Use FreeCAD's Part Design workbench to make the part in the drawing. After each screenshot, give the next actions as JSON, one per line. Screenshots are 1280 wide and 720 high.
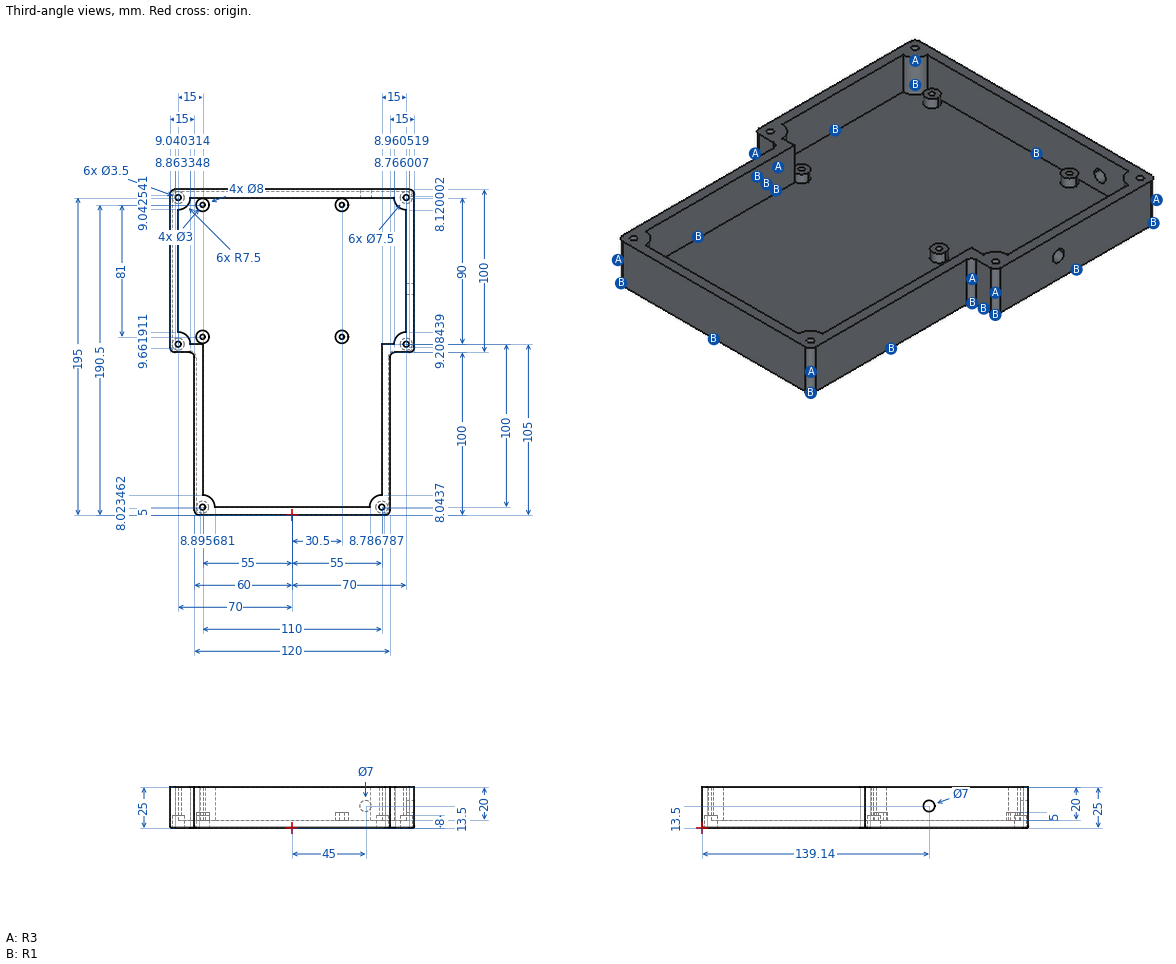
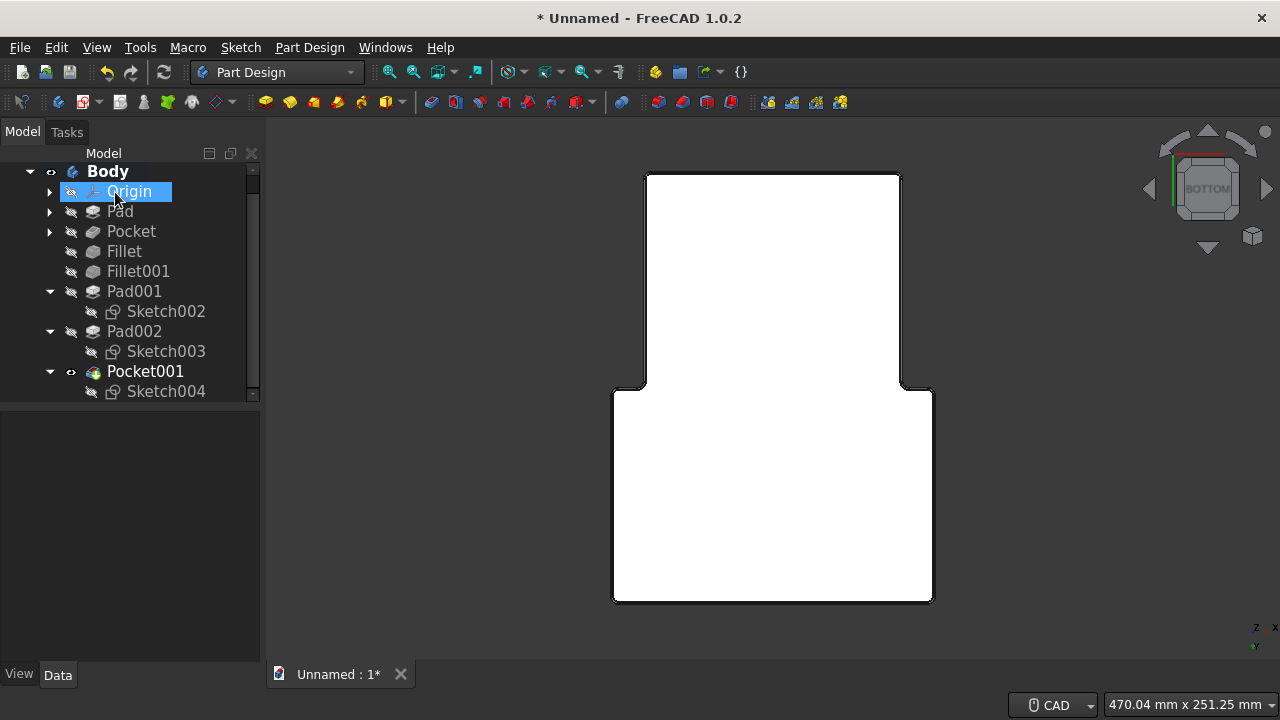
{"action": "left_click", "coordinate": [773, 448]}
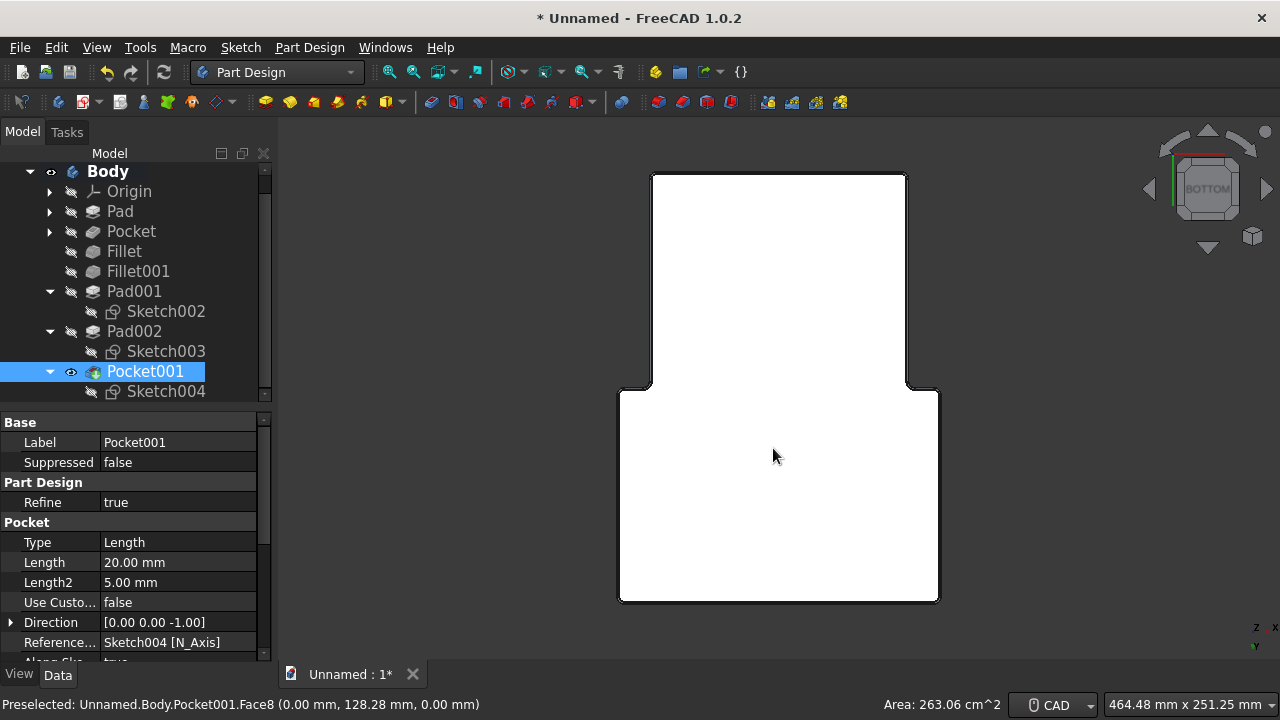
{"action": "left_click", "coordinate": [84, 102]}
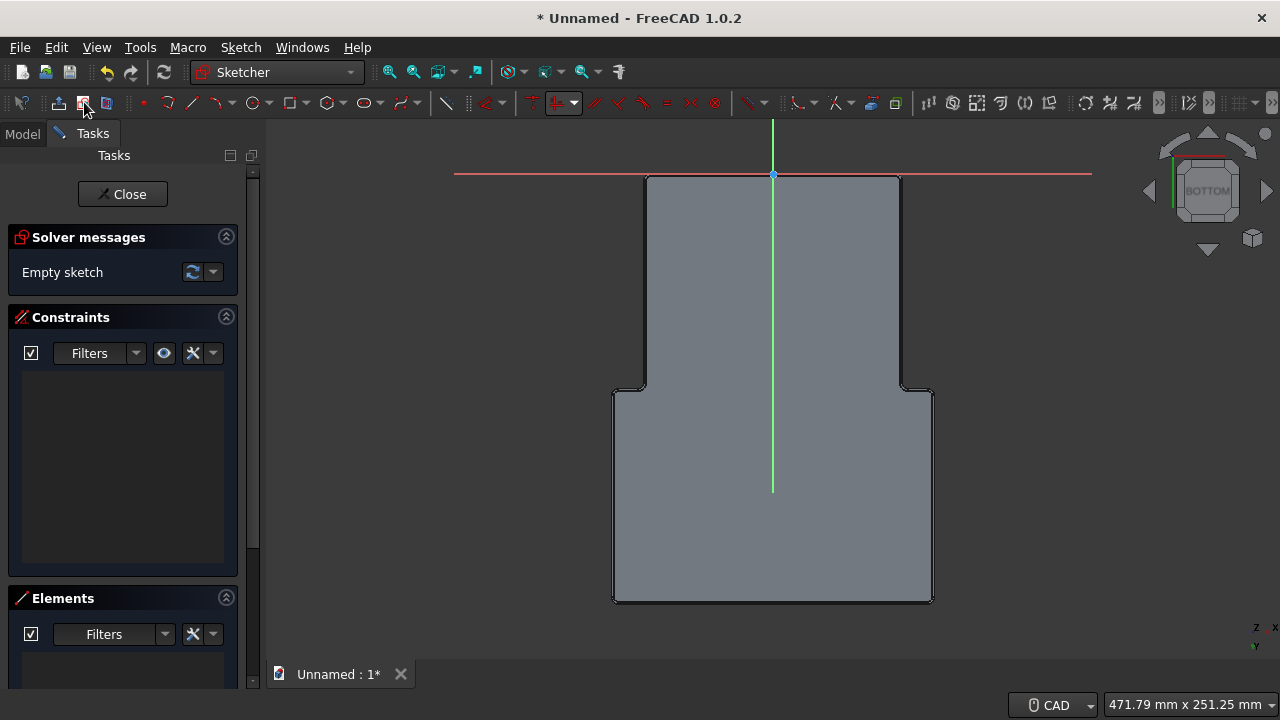
{"action": "key", "text": "g c"}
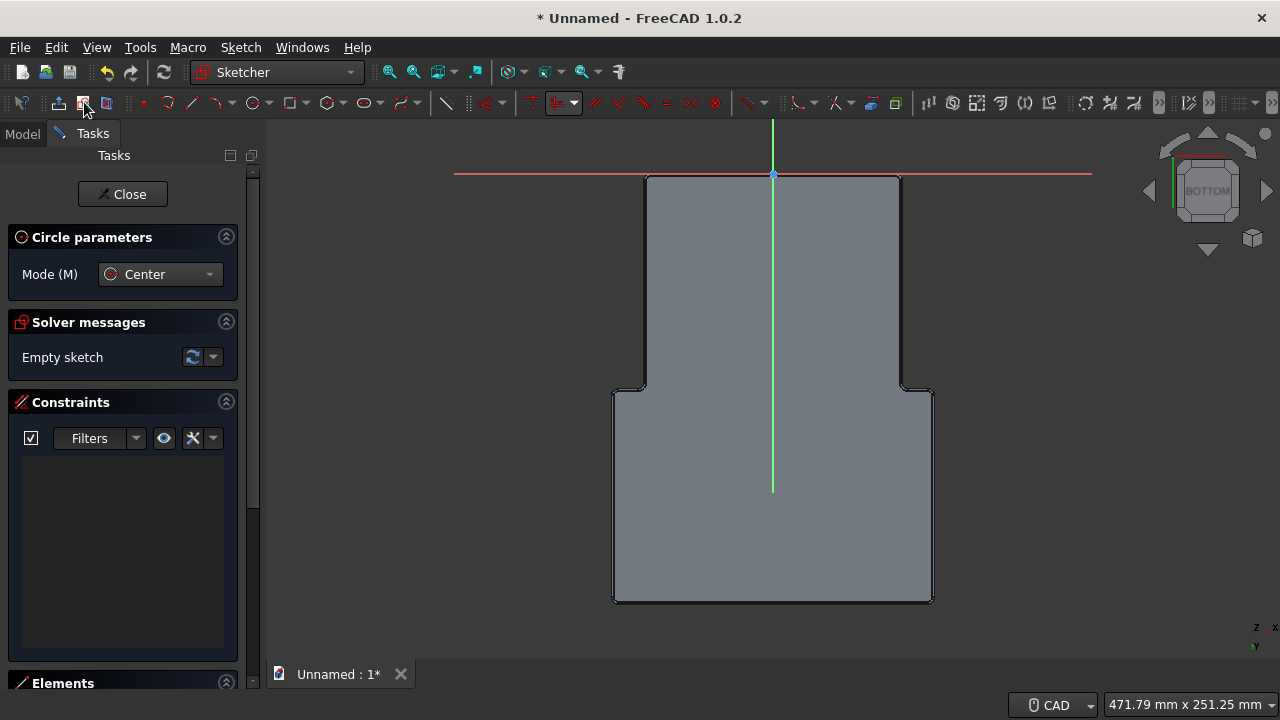
{"action": "scroll", "coordinate": [923, 593], "scroll_direction": "up", "scroll_amount": 6}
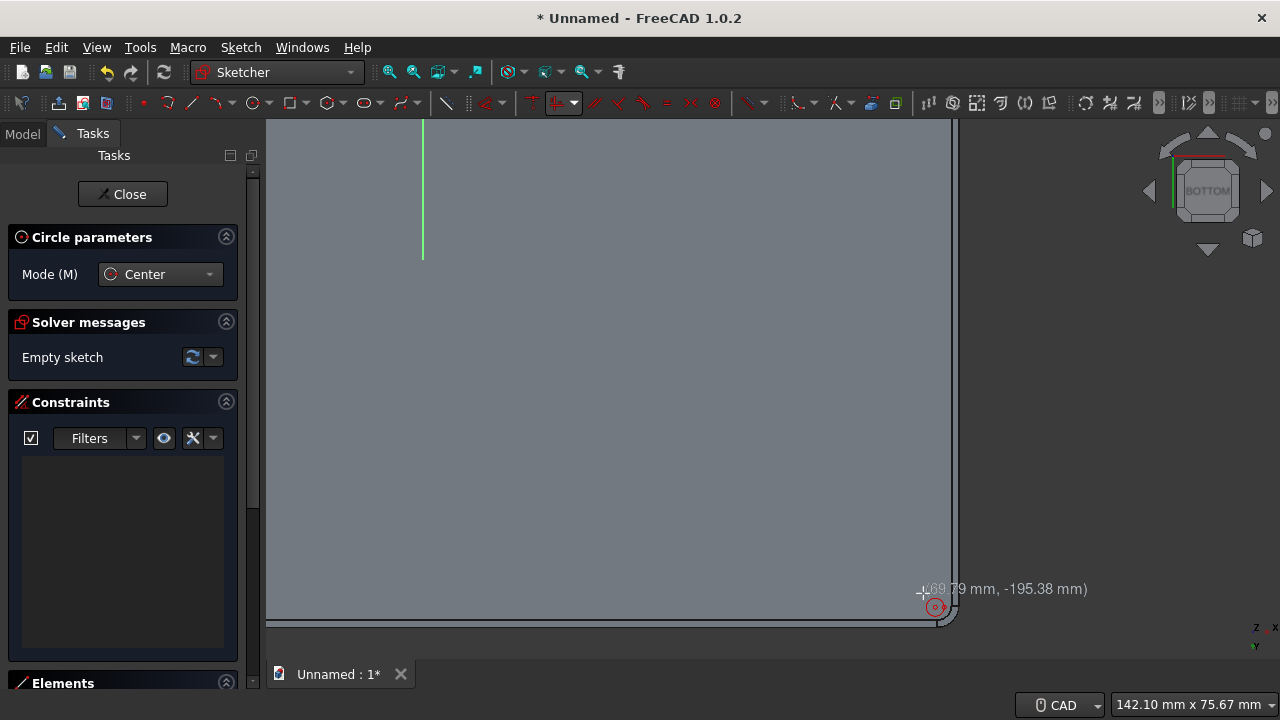
{"action": "left_click", "coordinate": [923, 592]}
{"action": "mouse_move", "coordinate": [942, 573]}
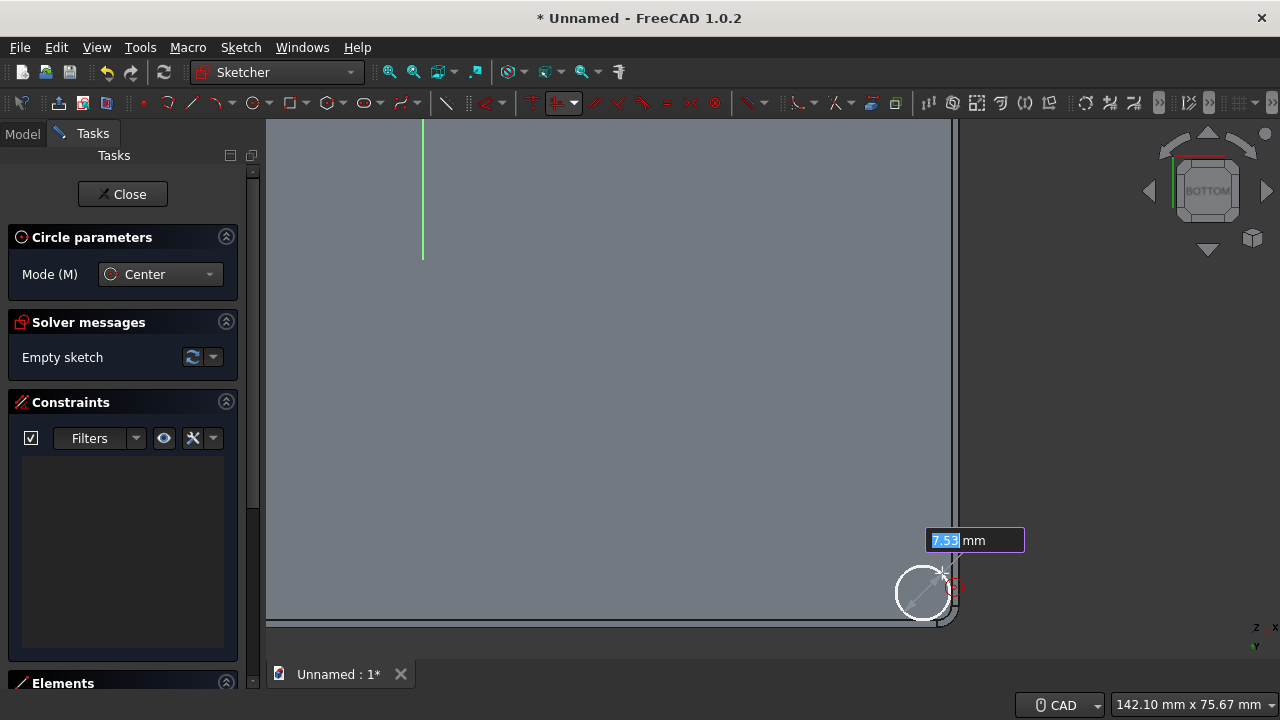
{"action": "type", "text": "7.5"}
{"action": "key", "text": "Return"}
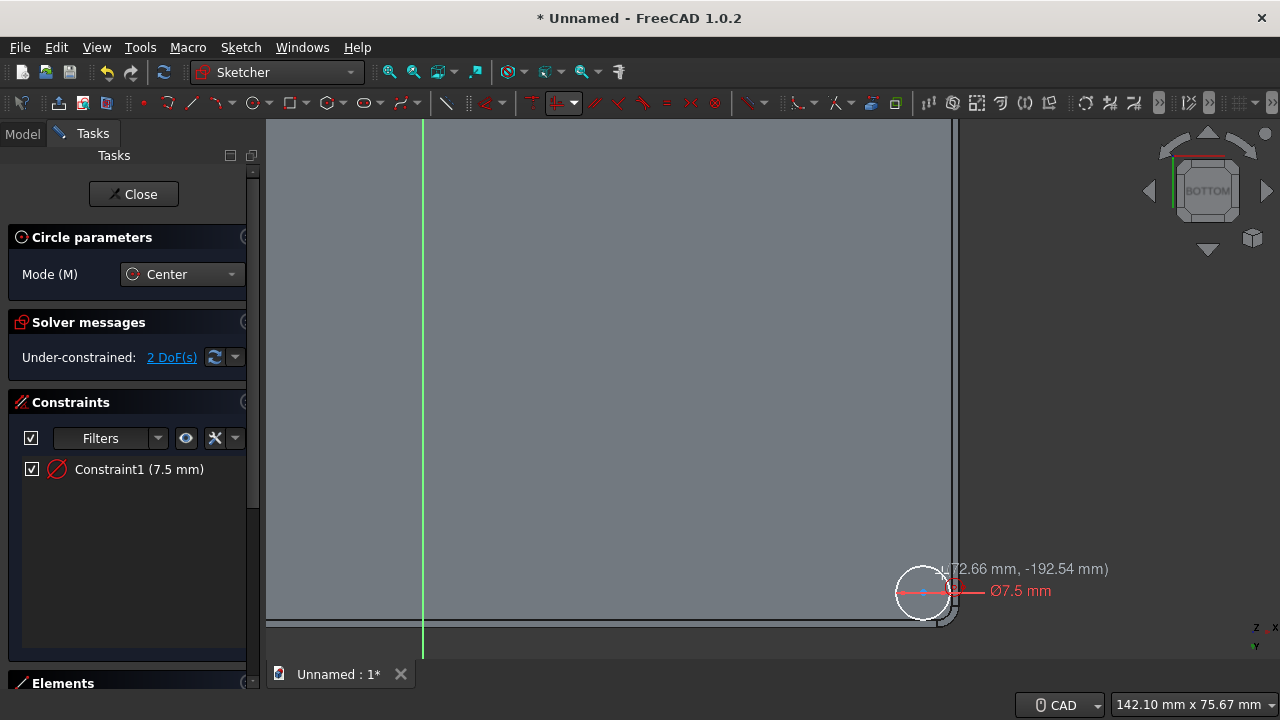
{"action": "scroll", "coordinate": [796, 546], "scroll_direction": "down", "scroll_amount": 7}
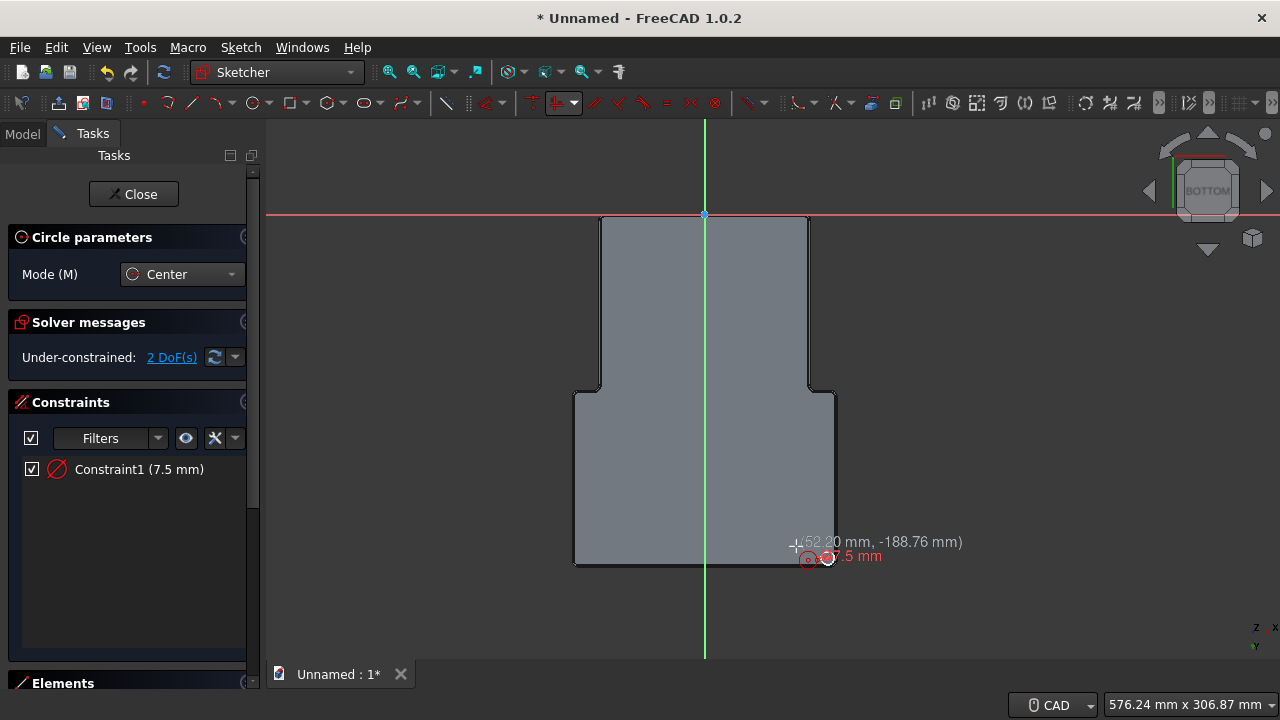
{"action": "scroll", "coordinate": [828, 399], "scroll_direction": "up", "scroll_amount": 7}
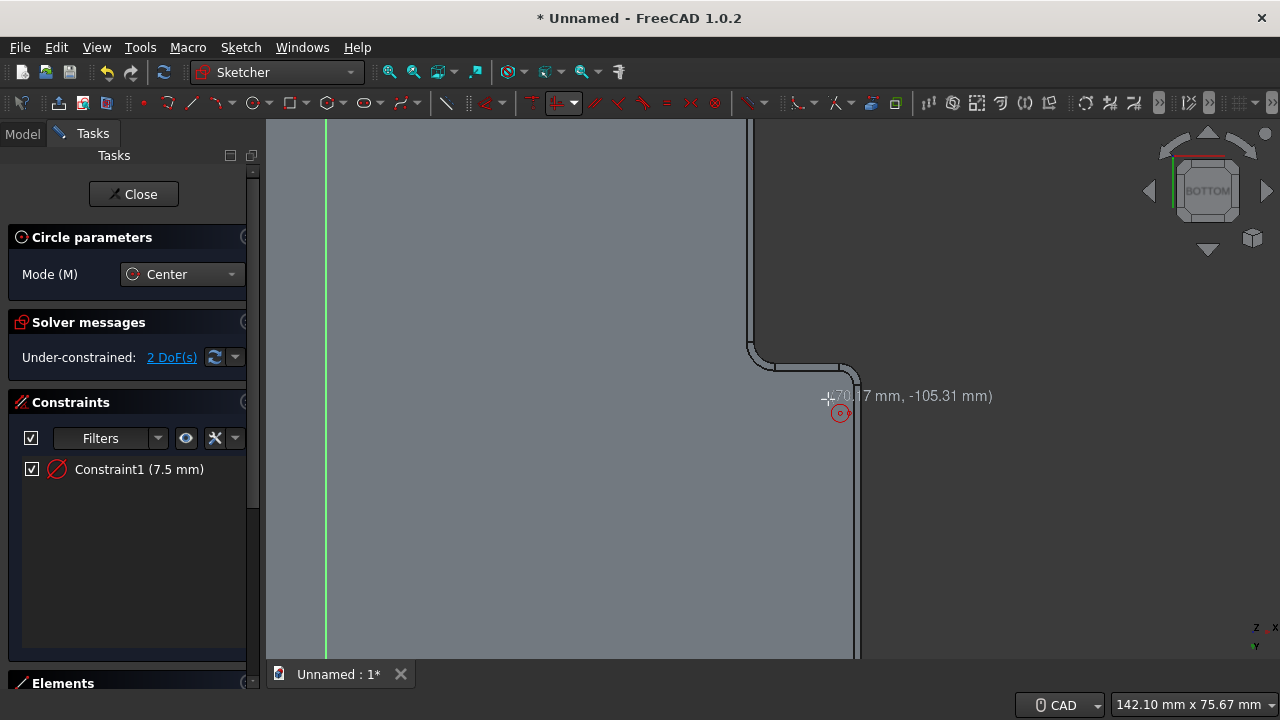
{"action": "left_click", "coordinate": [825, 399]}
{"action": "mouse_move", "coordinate": [844, 380]}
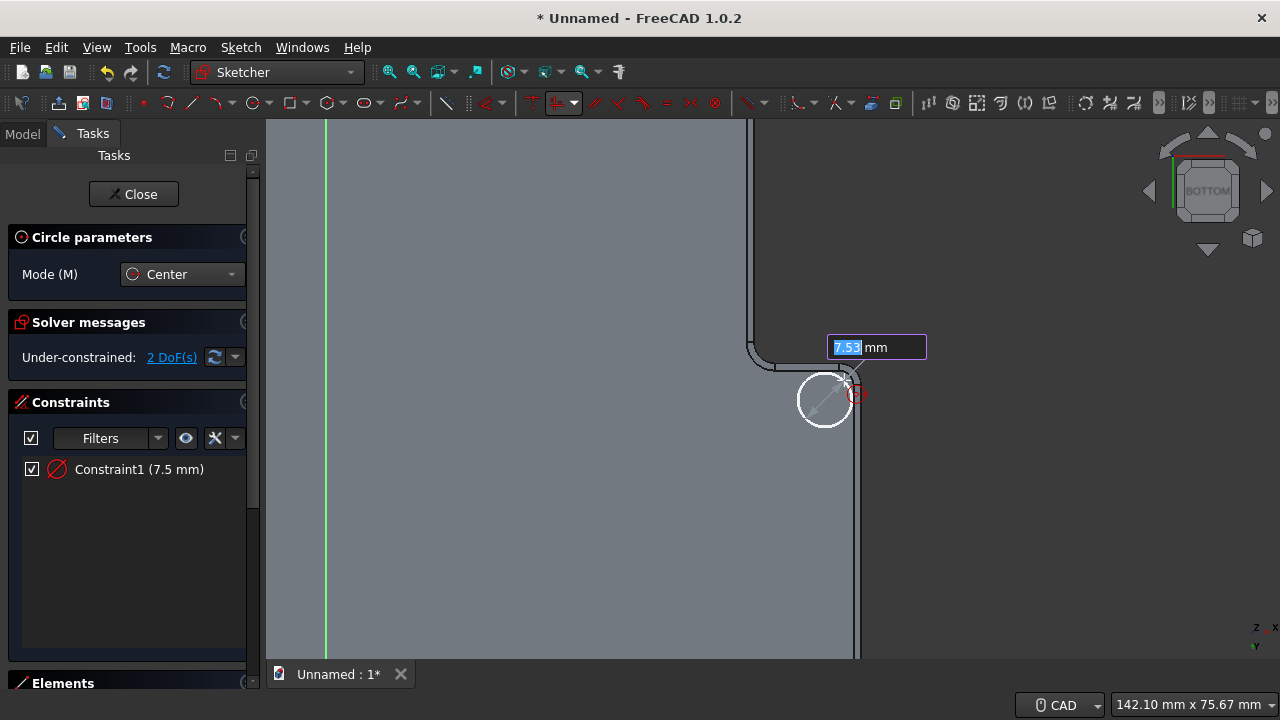
{"action": "type", "text": "7.5"}
{"action": "key", "text": "Return"}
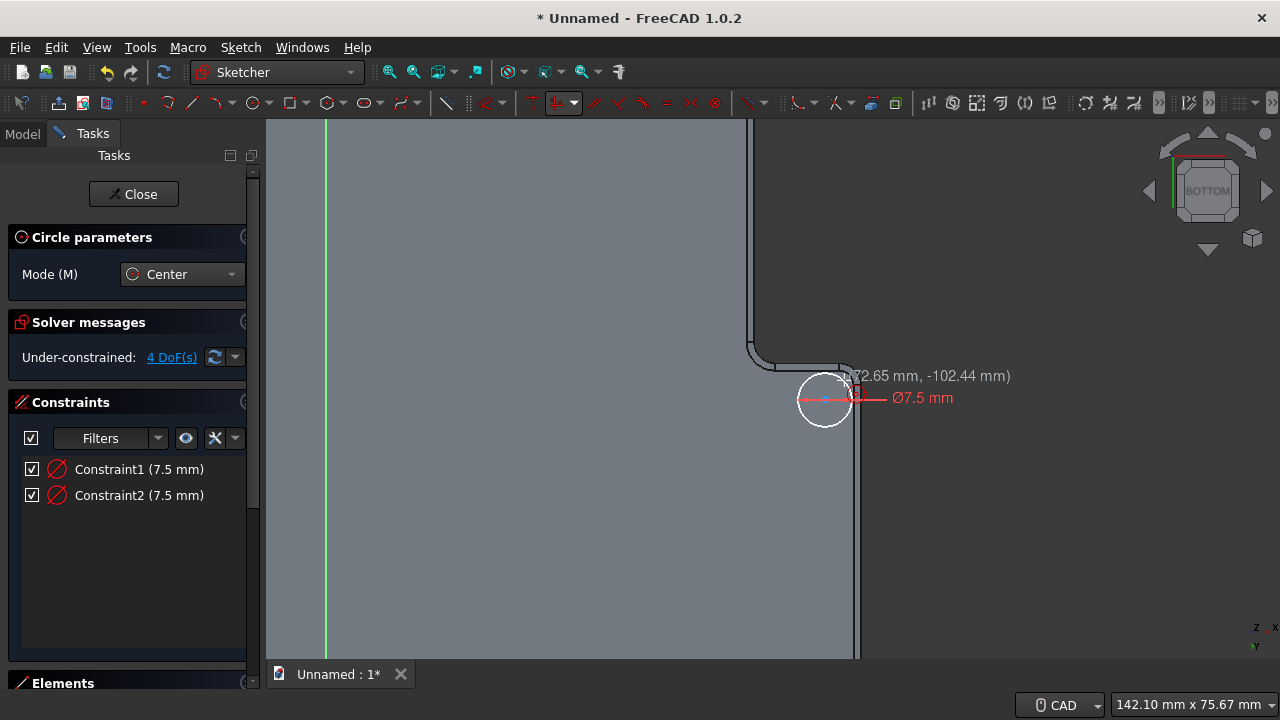
{"action": "scroll", "coordinate": [829, 399], "scroll_direction": "down", "scroll_amount": 7}